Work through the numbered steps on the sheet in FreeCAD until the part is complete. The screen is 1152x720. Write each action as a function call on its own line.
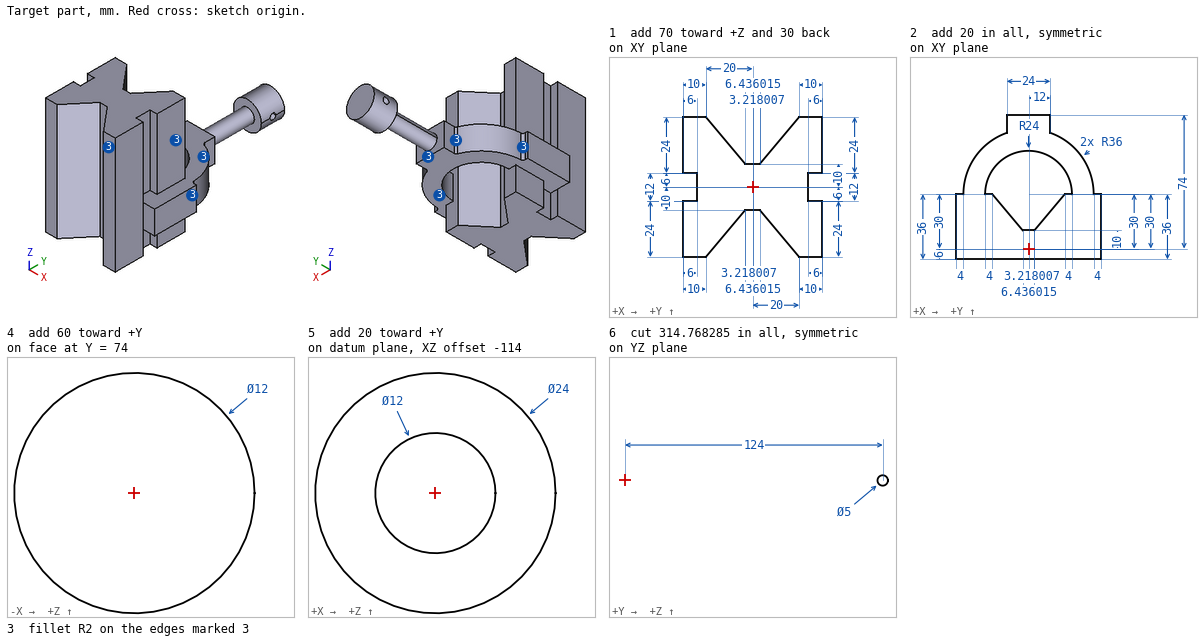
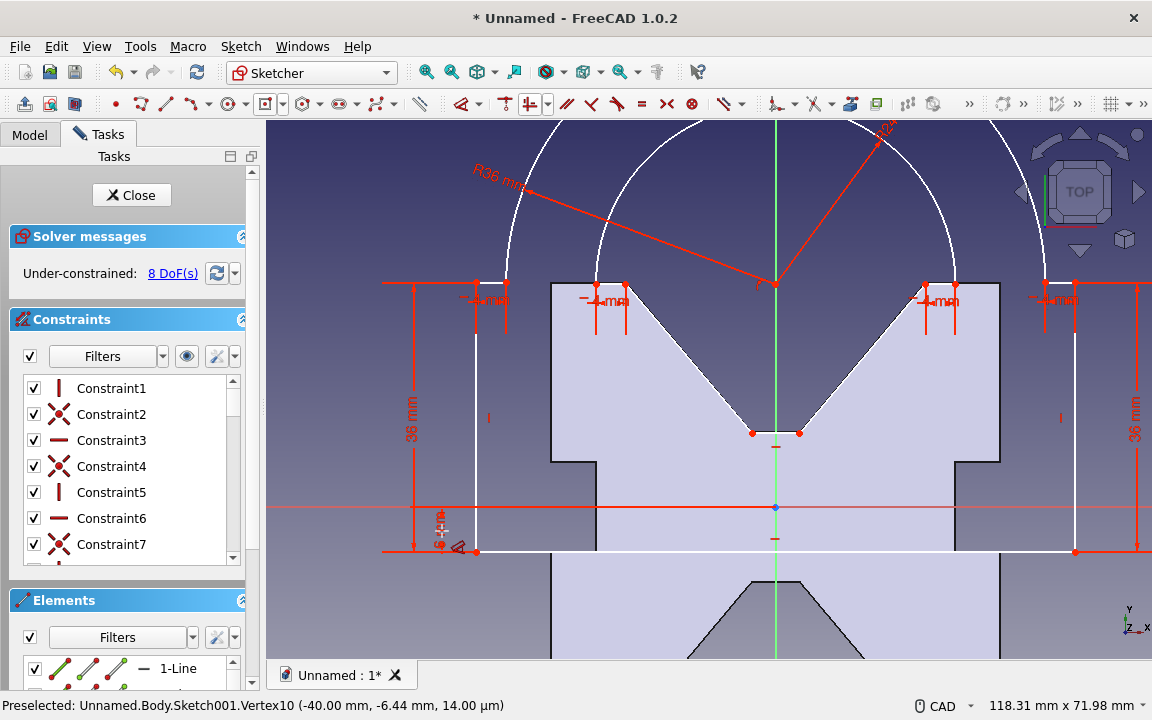
scroll(476, 556, down, 3)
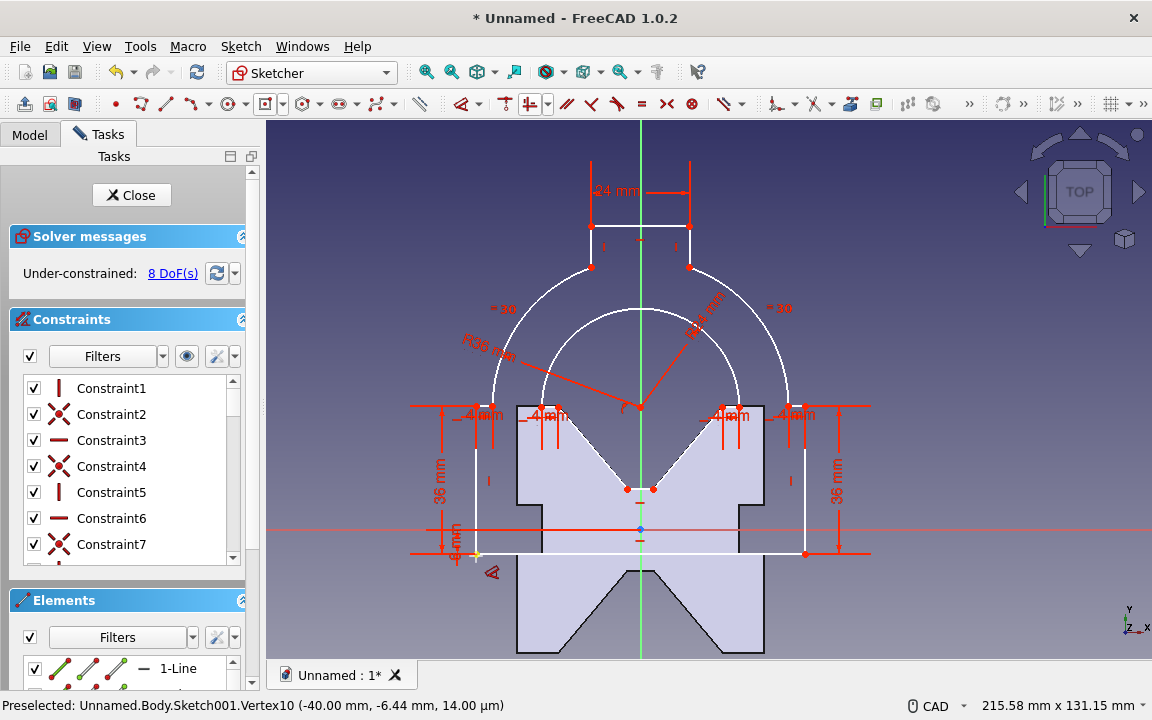
click(690, 268)
click(665, 588)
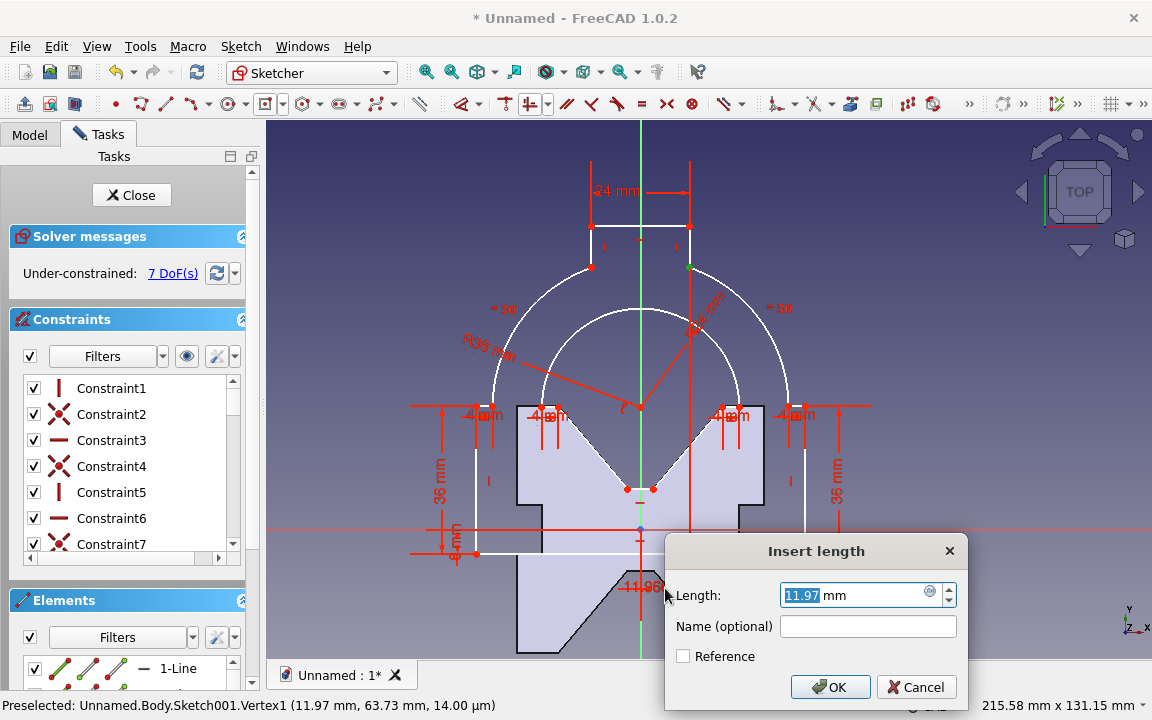
text(12)
key(Return)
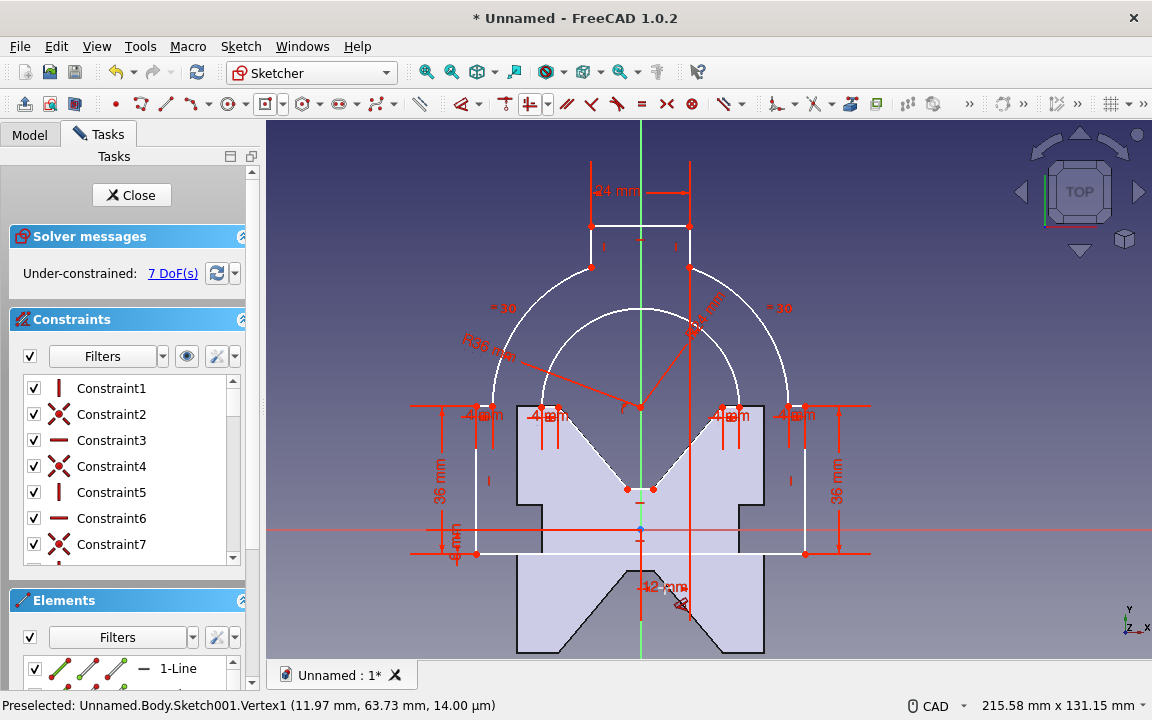
click(690, 226)
click(724, 448)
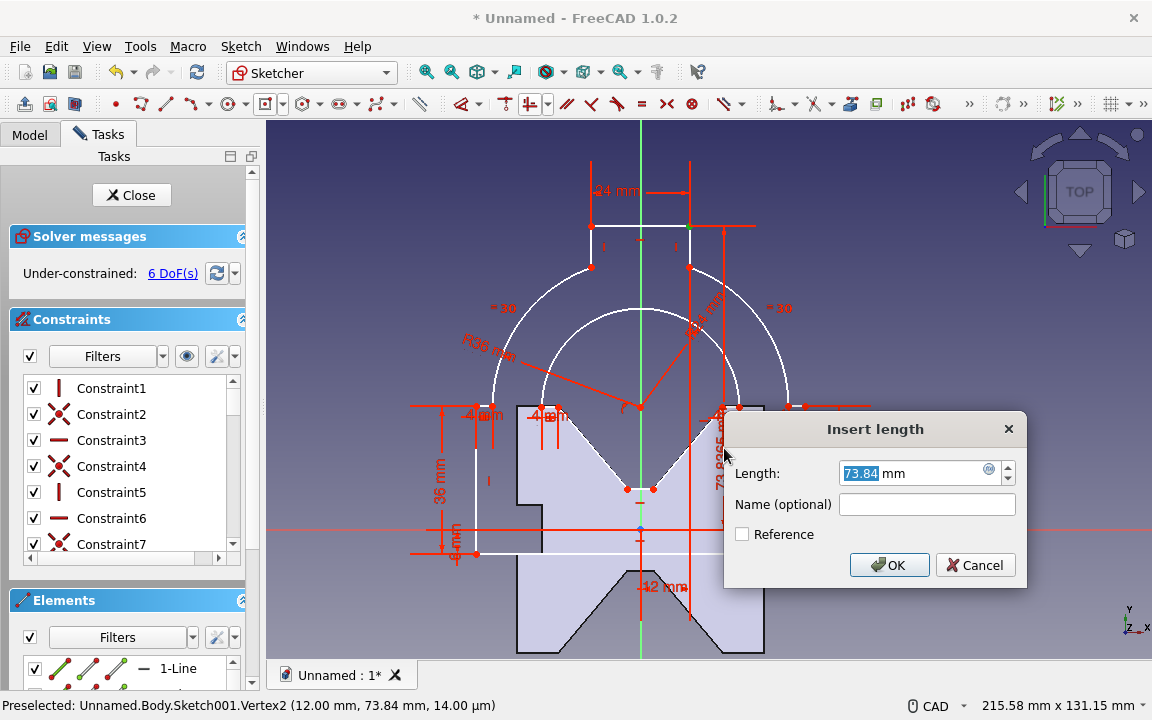
text(74)
key(Return)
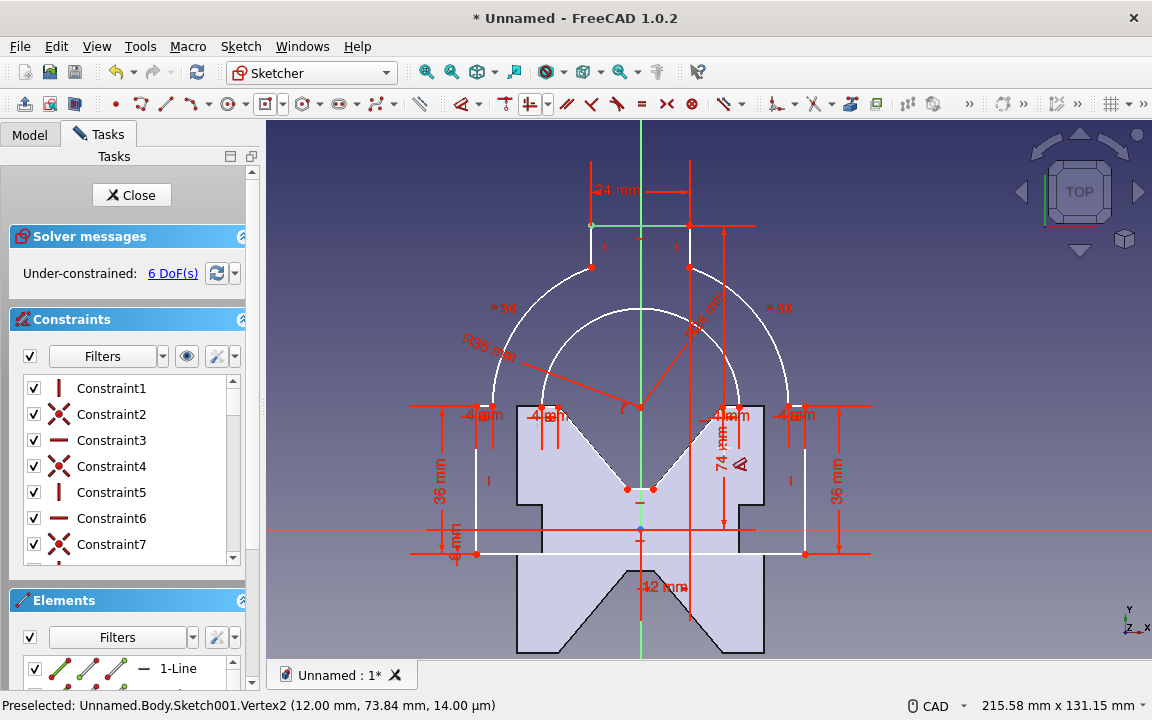
click(739, 407)
click(773, 511)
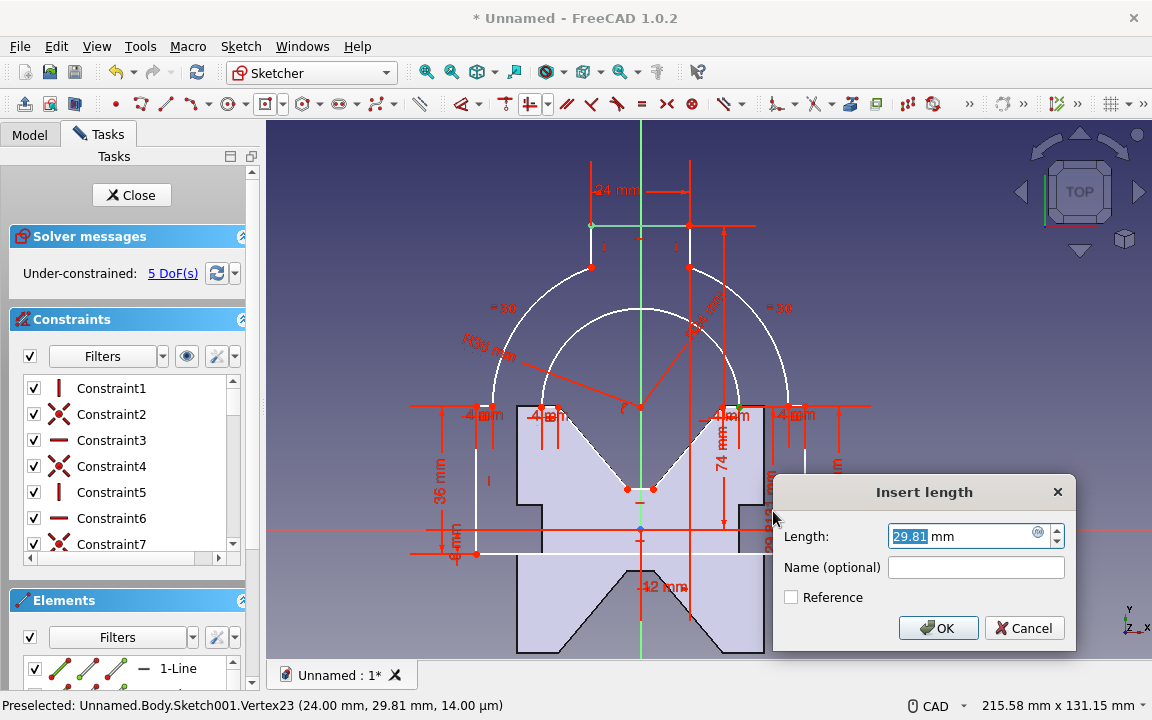
text(30)
key(Return)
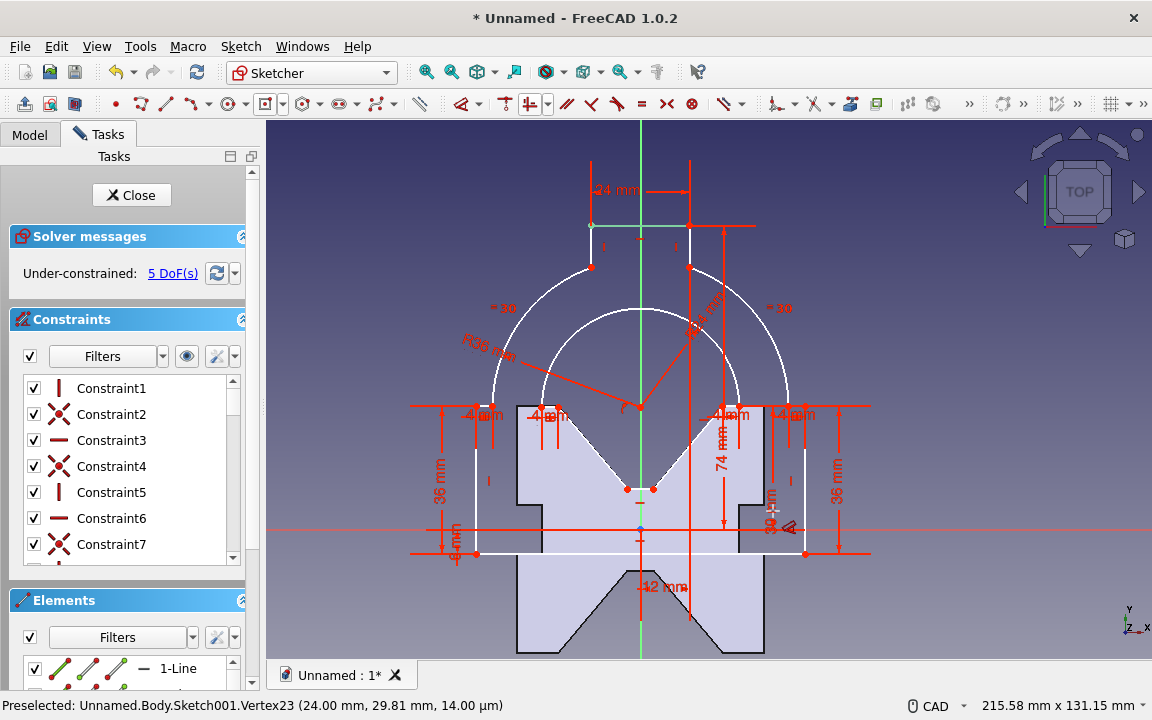
click(654, 489)
click(688, 509)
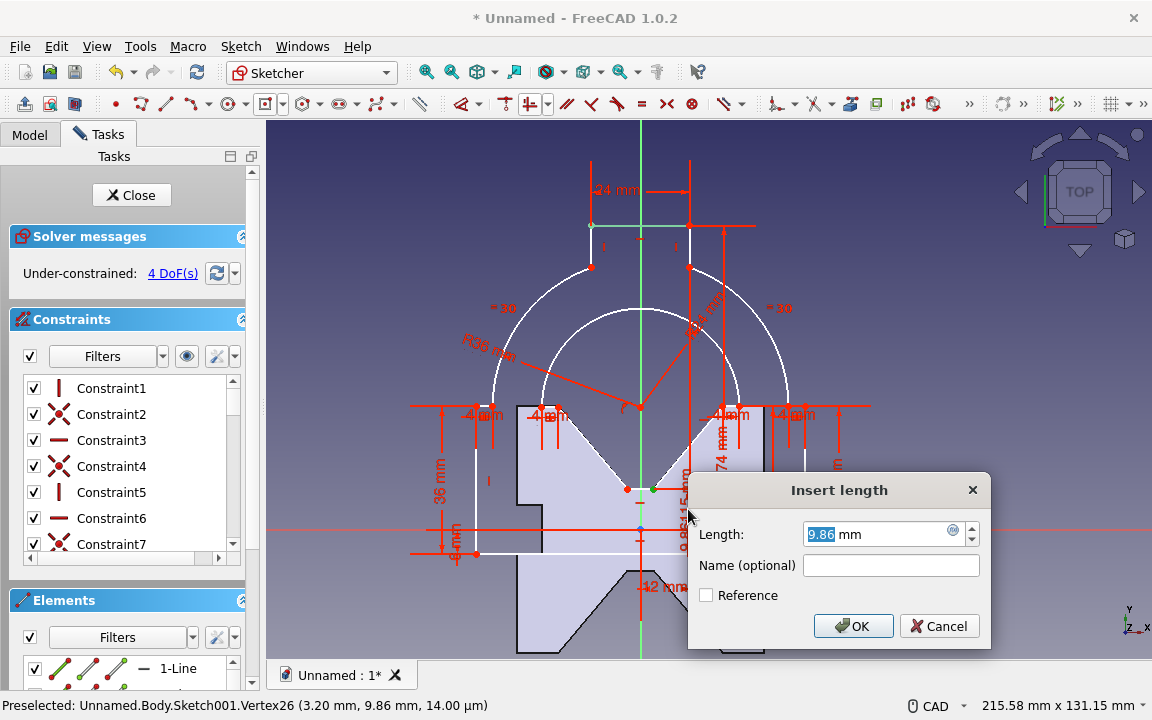
text(10)
key(Return)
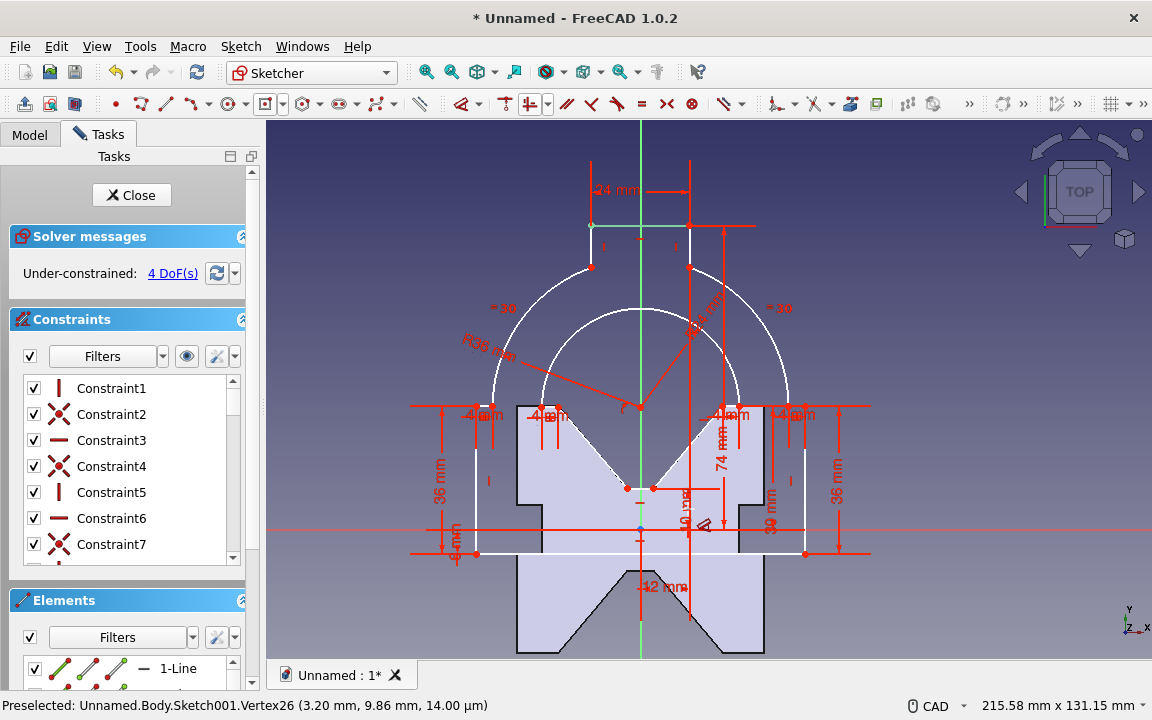
click(558, 407)
click(524, 468)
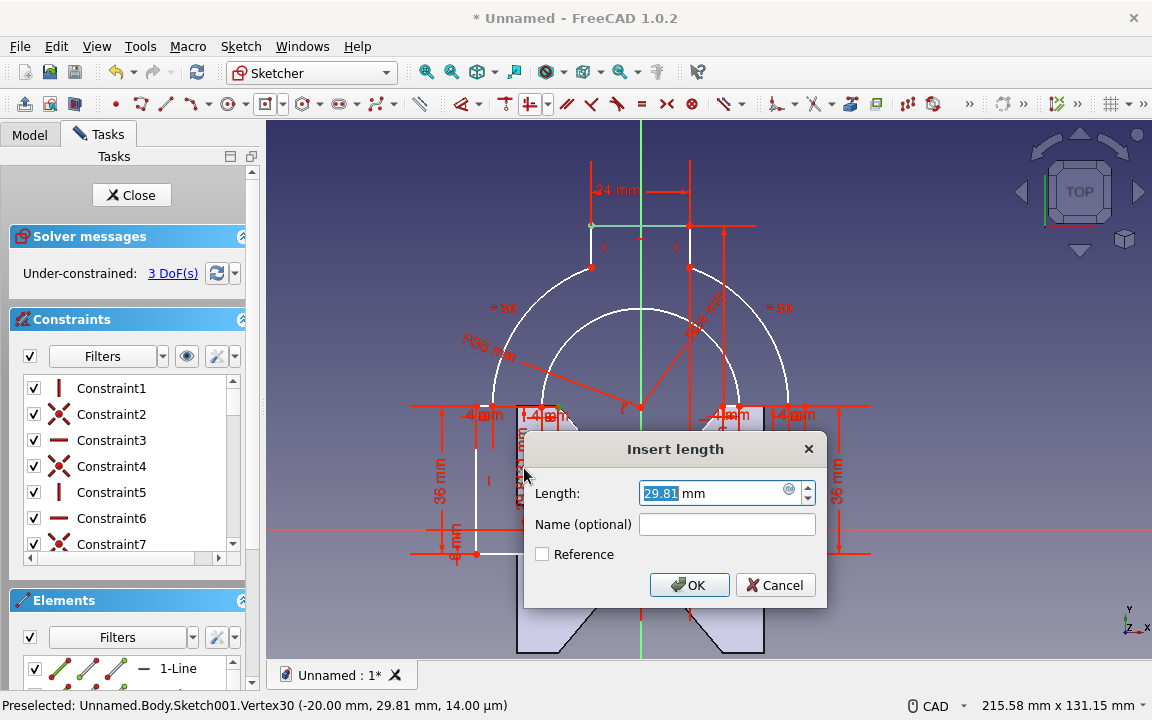
text(30)
key(Return)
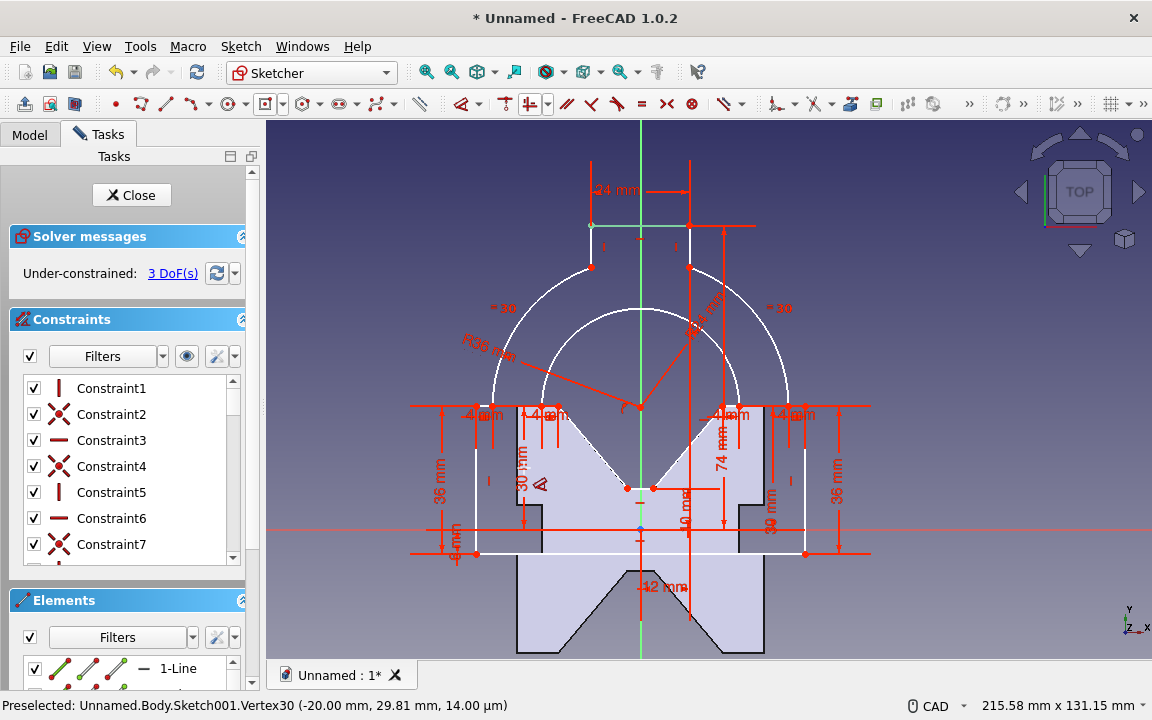
click(641, 407)
click(607, 440)